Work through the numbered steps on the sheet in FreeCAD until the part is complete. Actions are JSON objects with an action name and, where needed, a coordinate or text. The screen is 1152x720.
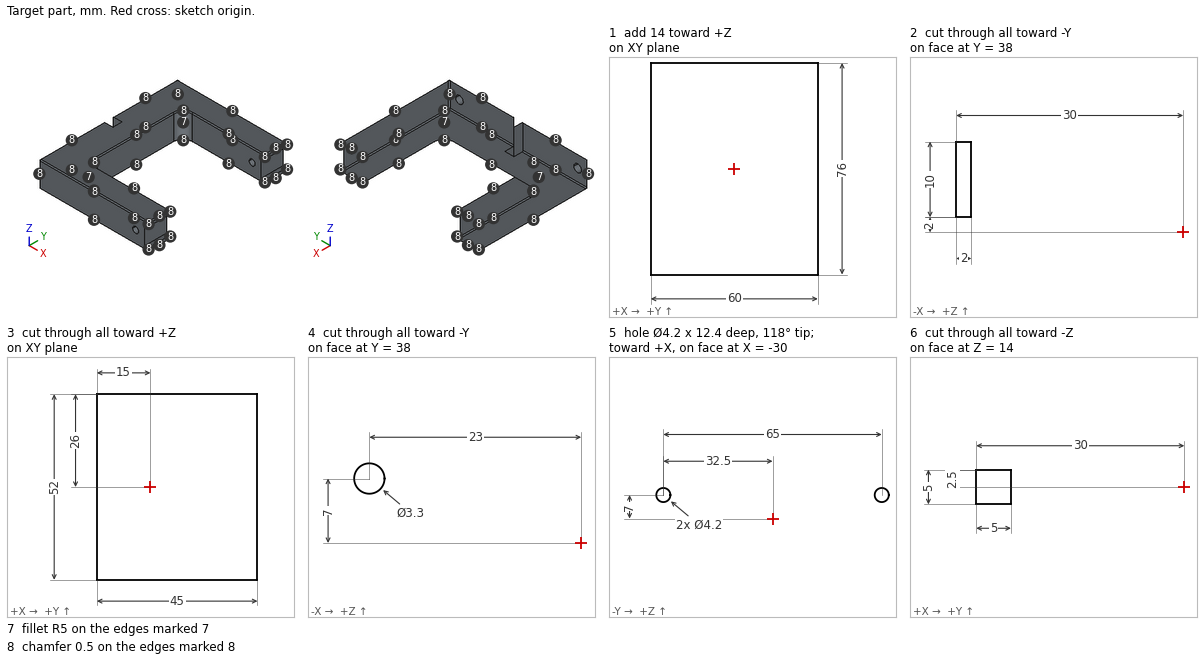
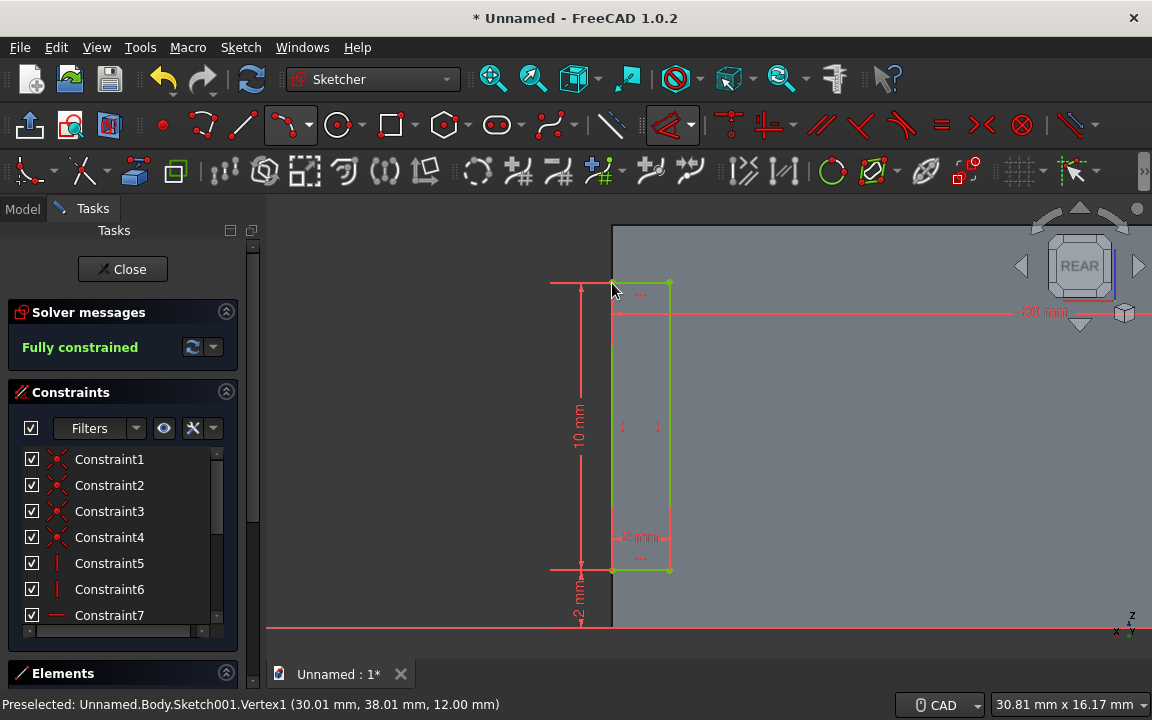
{"action": "left_click", "coordinate": [123, 269]}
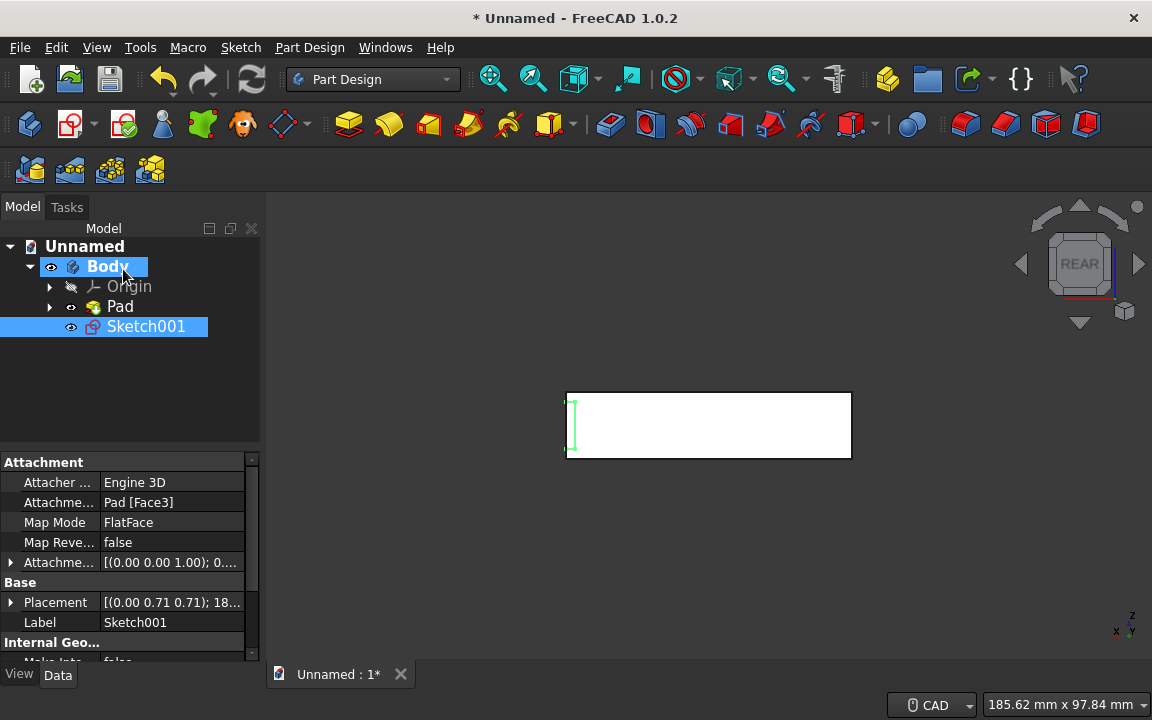
{"action": "left_click", "coordinate": [612, 124]}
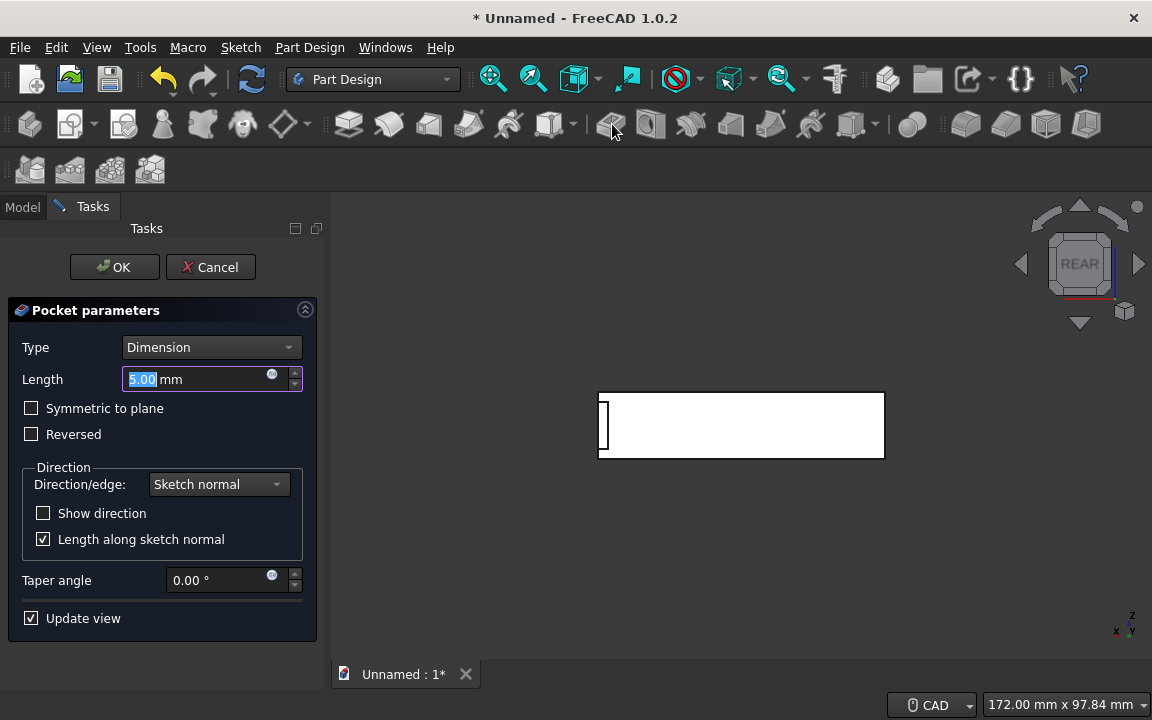
{"action": "left_click", "coordinate": [212, 348]}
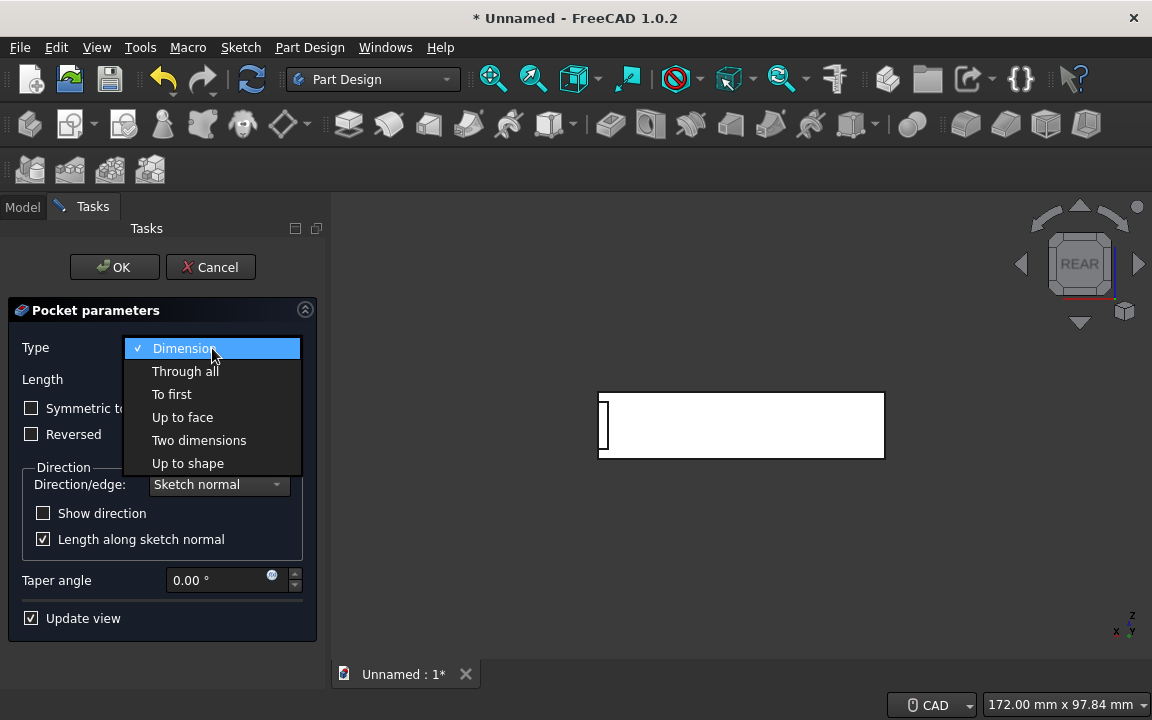
{"action": "left_click", "coordinate": [212, 372]}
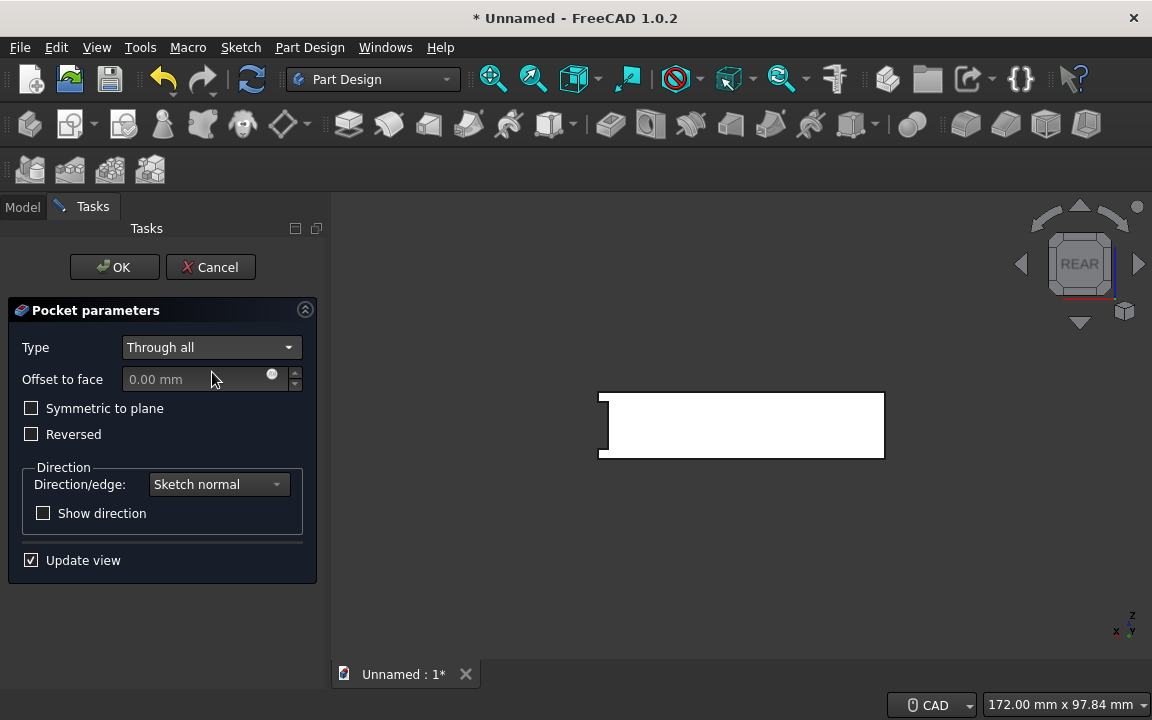
{"action": "left_click", "coordinate": [115, 267]}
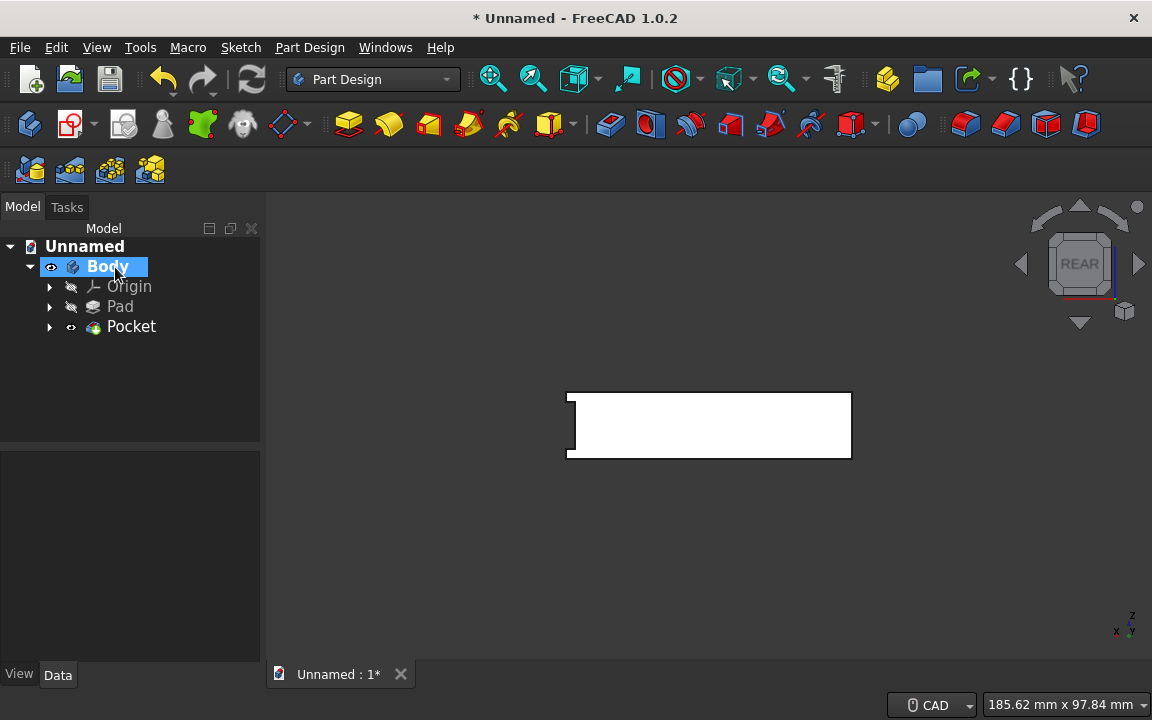
{"action": "left_click", "coordinate": [494, 80]}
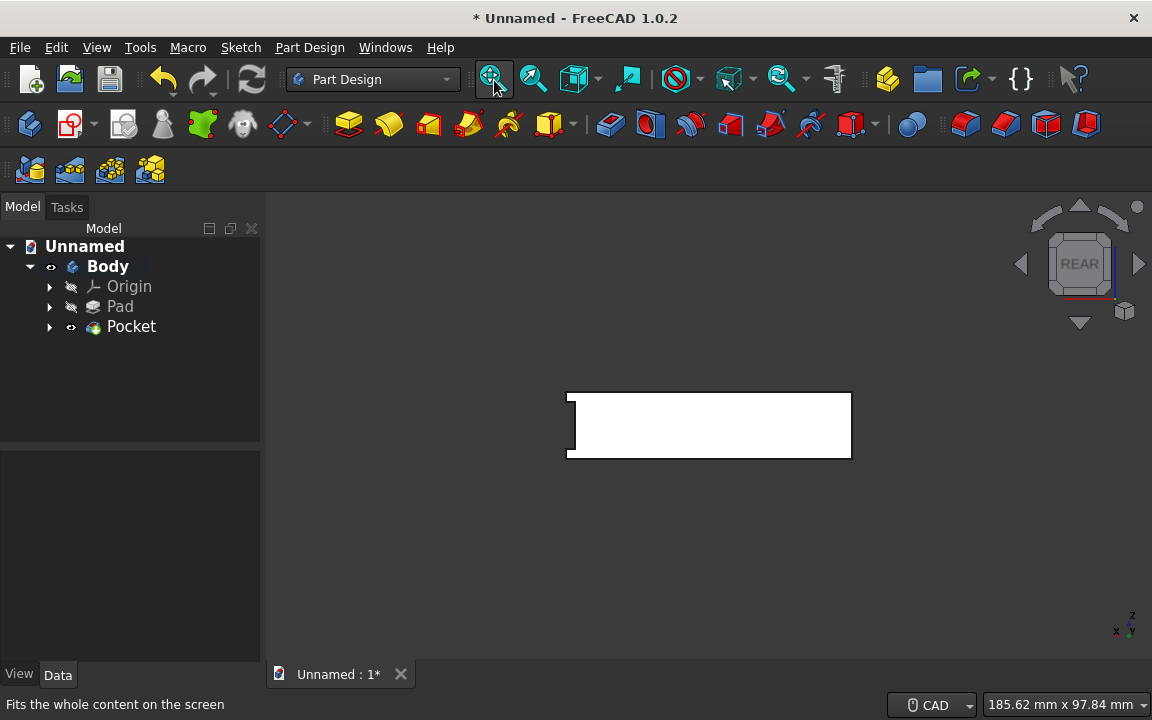
{"action": "left_click", "coordinate": [70, 124]}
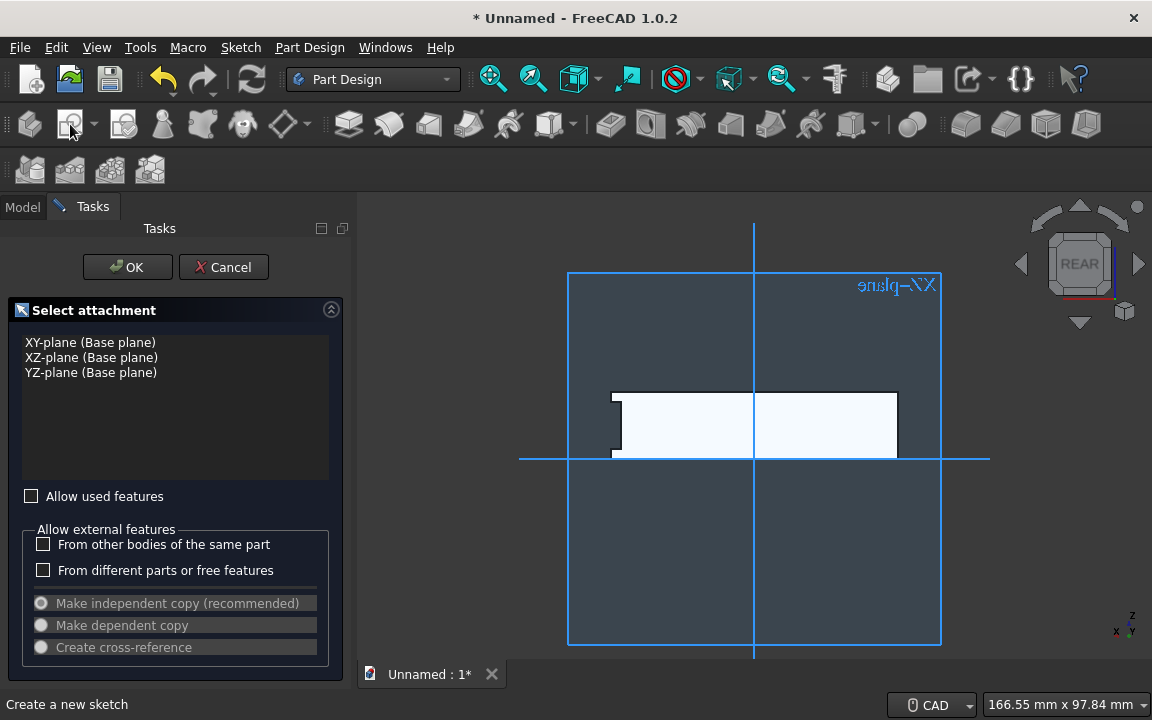
{"action": "left_click", "coordinate": [82, 342]}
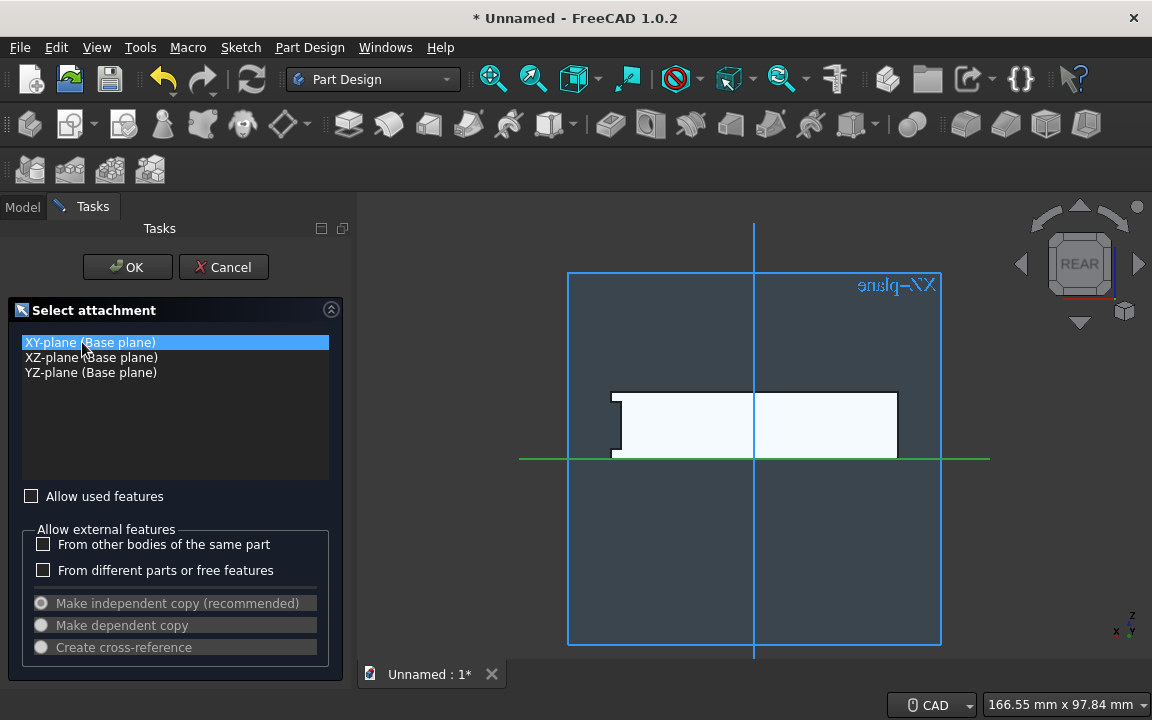
{"action": "left_click", "coordinate": [128, 267]}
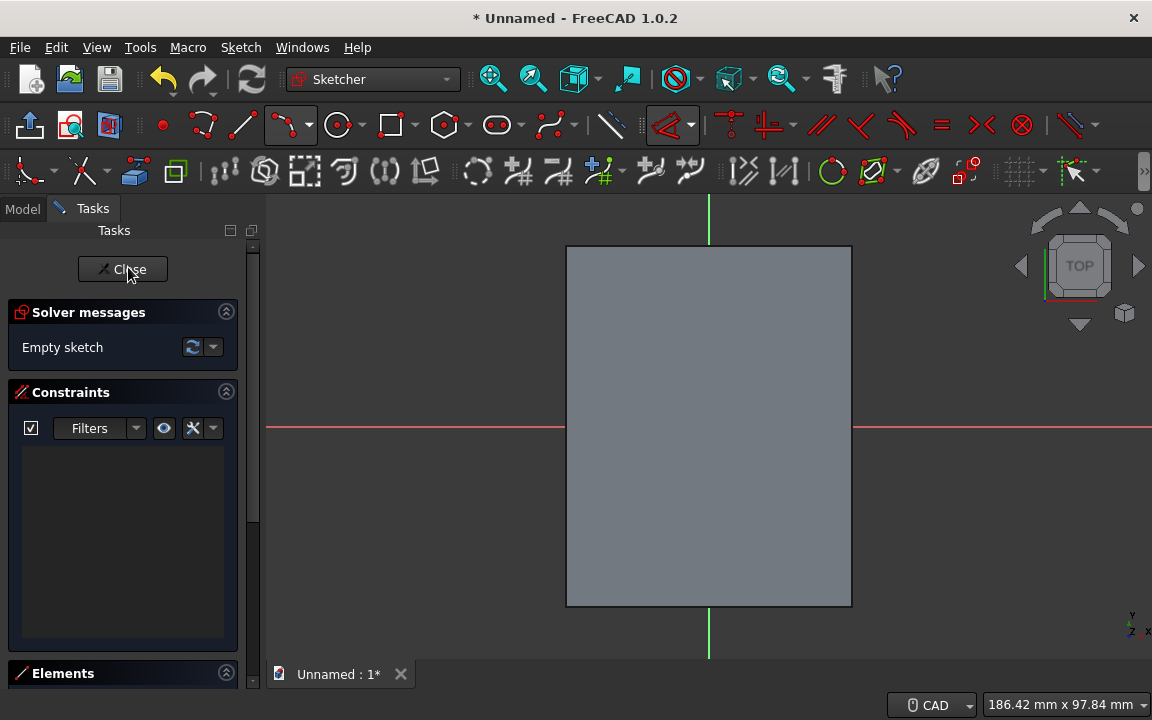
{"action": "key", "text": "q s"}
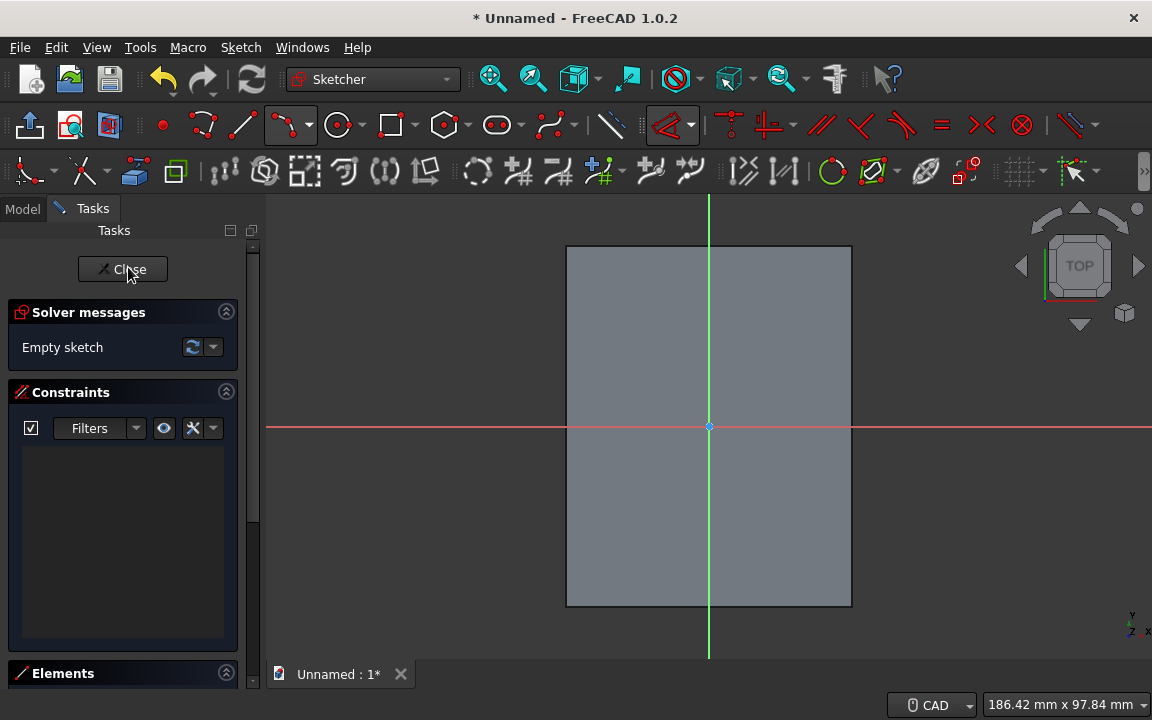
{"action": "key", "text": "g r"}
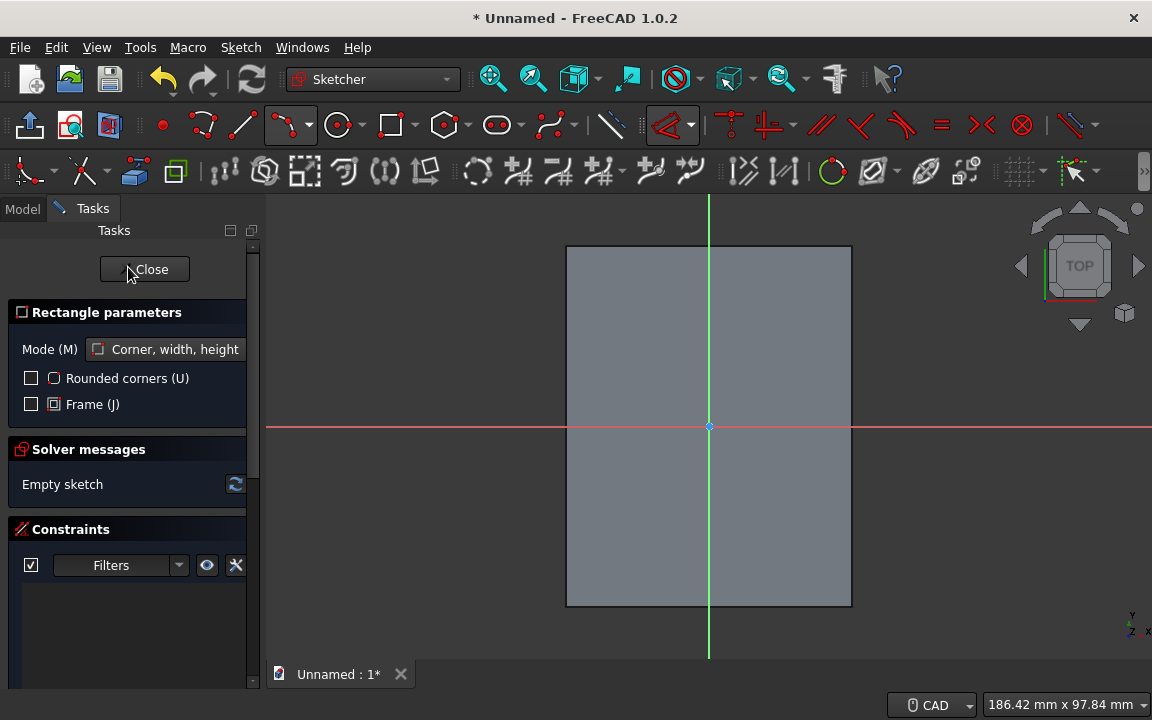
{"action": "left_click", "coordinate": [638, 303]}
{"action": "left_click", "coordinate": [852, 550]}
{"action": "key", "text": "Escape"}